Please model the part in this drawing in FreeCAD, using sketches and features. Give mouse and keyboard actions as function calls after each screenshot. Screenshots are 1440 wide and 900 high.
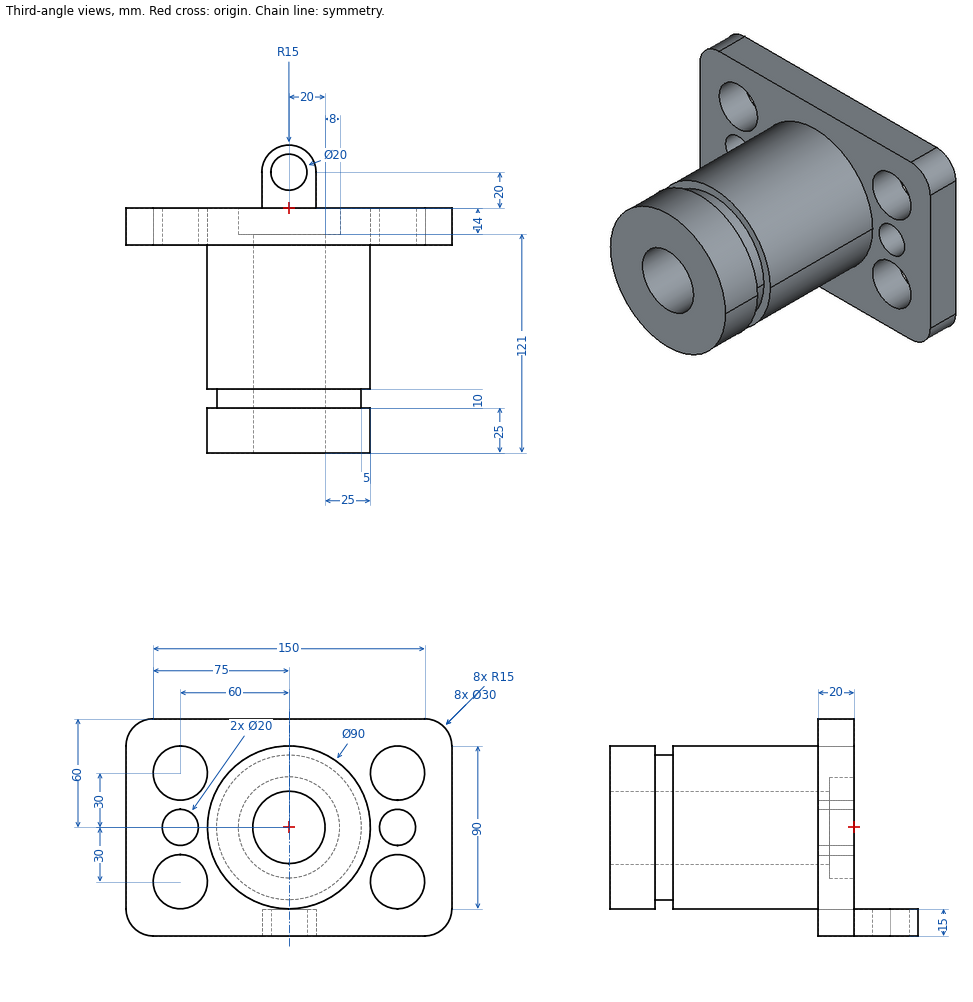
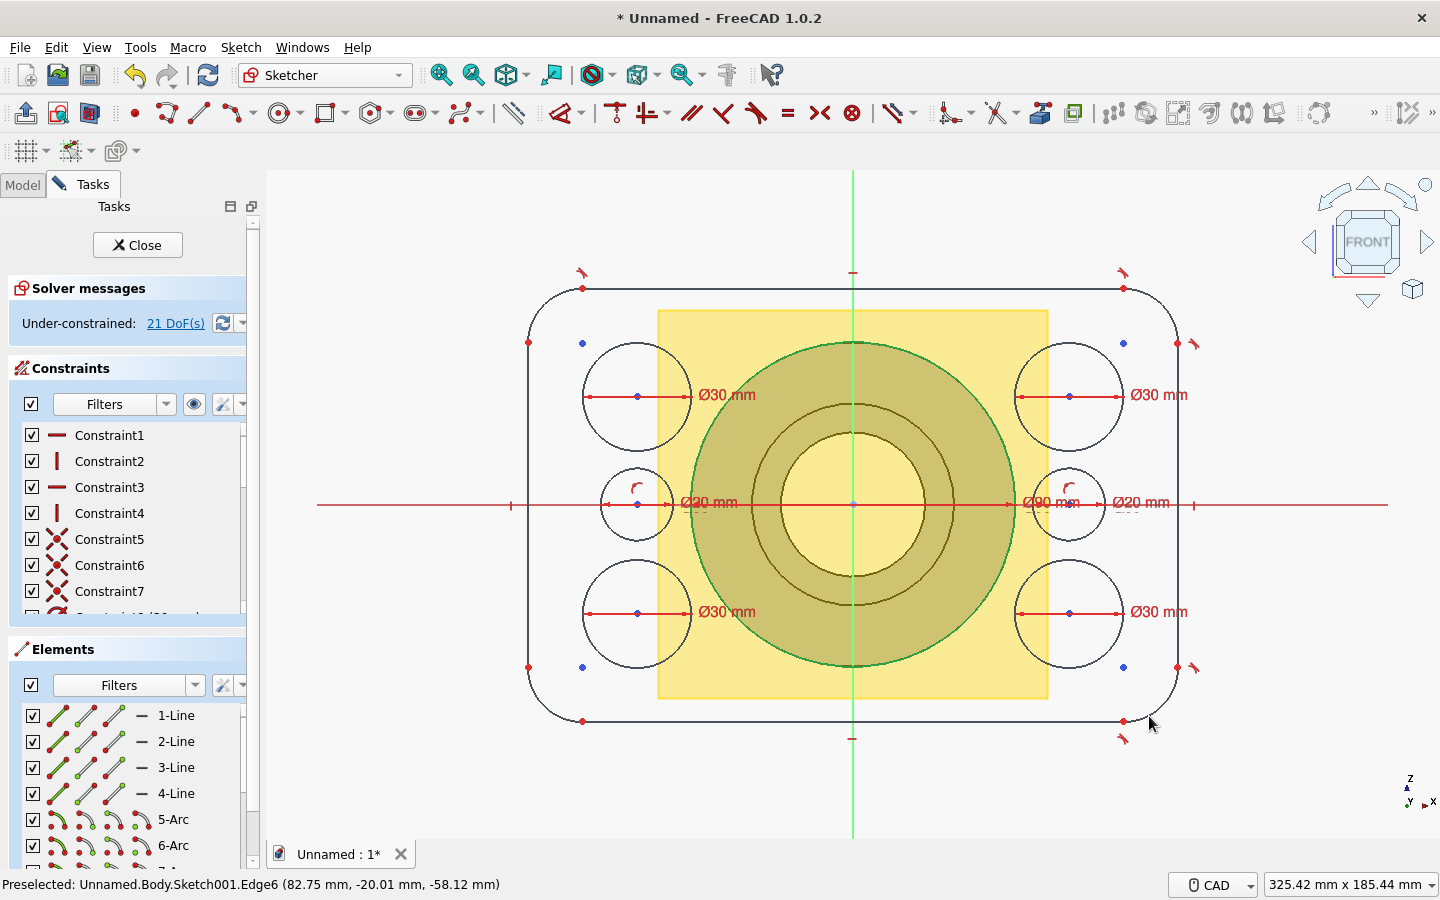
click(961, 722)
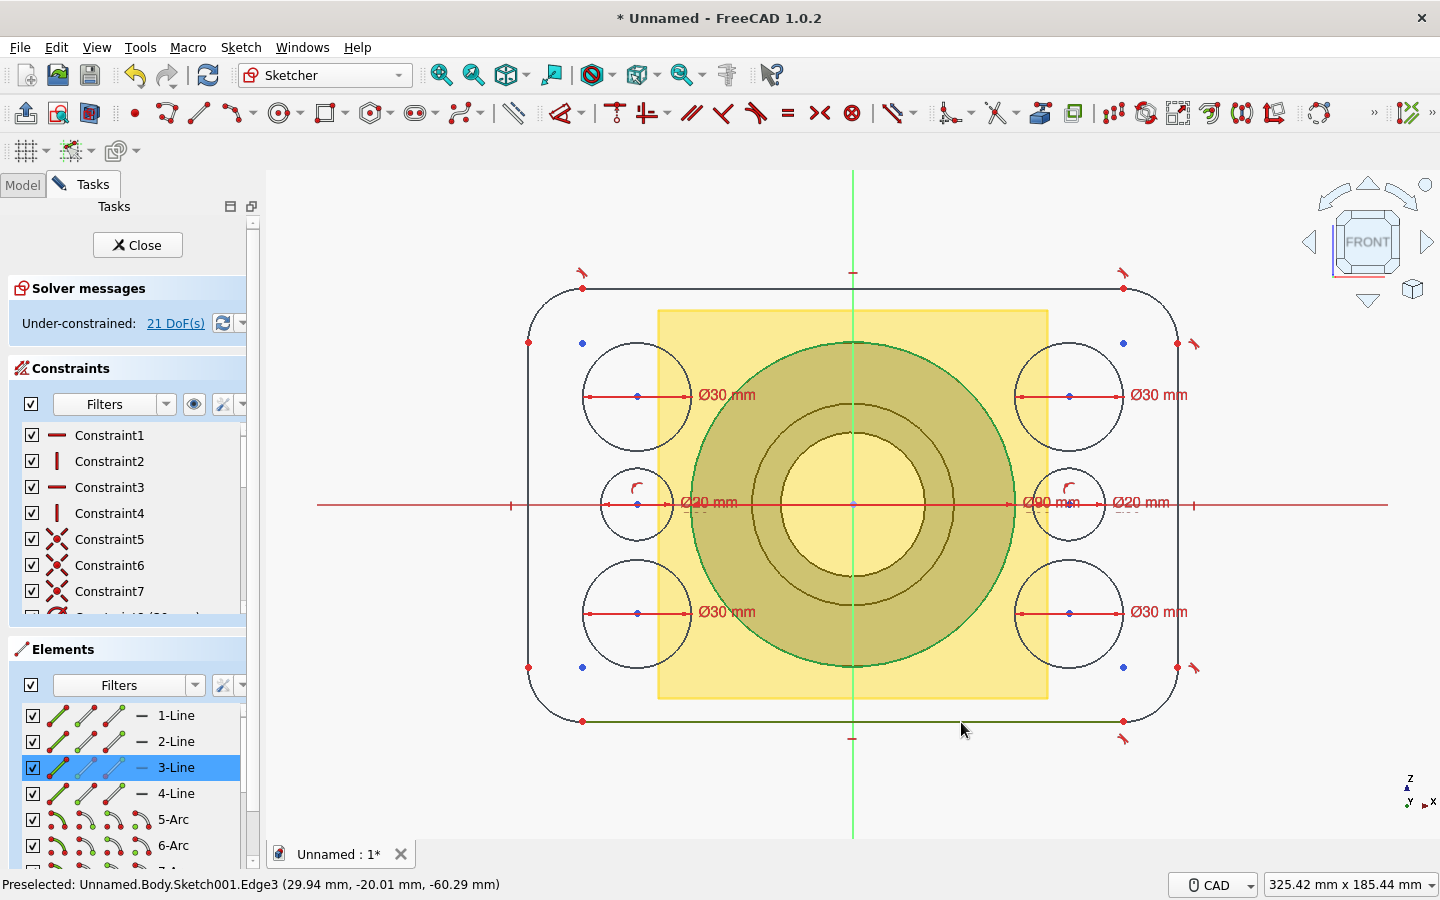
click(534, 692)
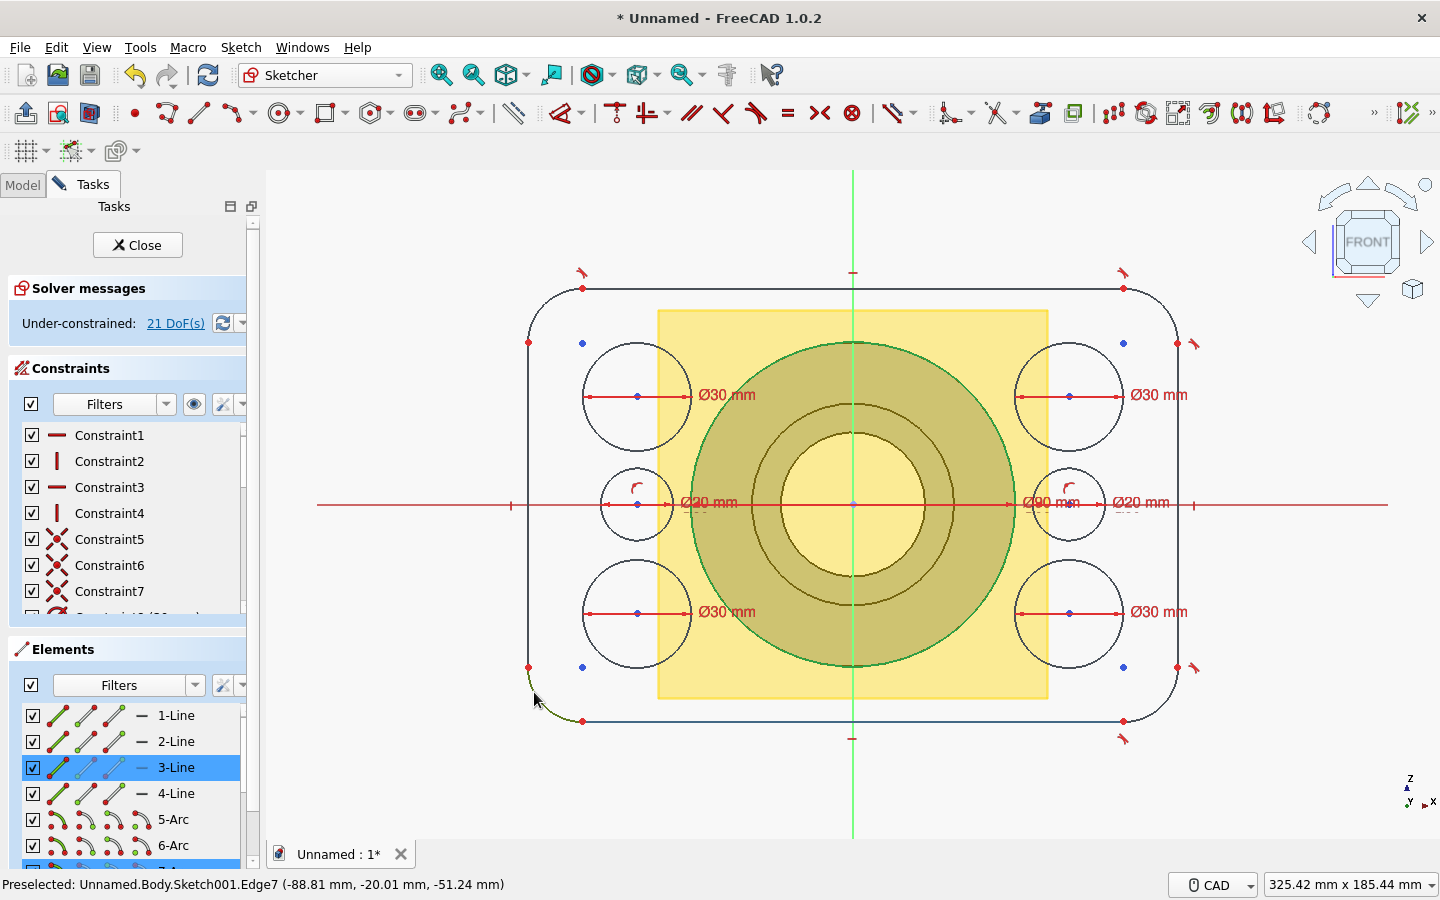
click(756, 114)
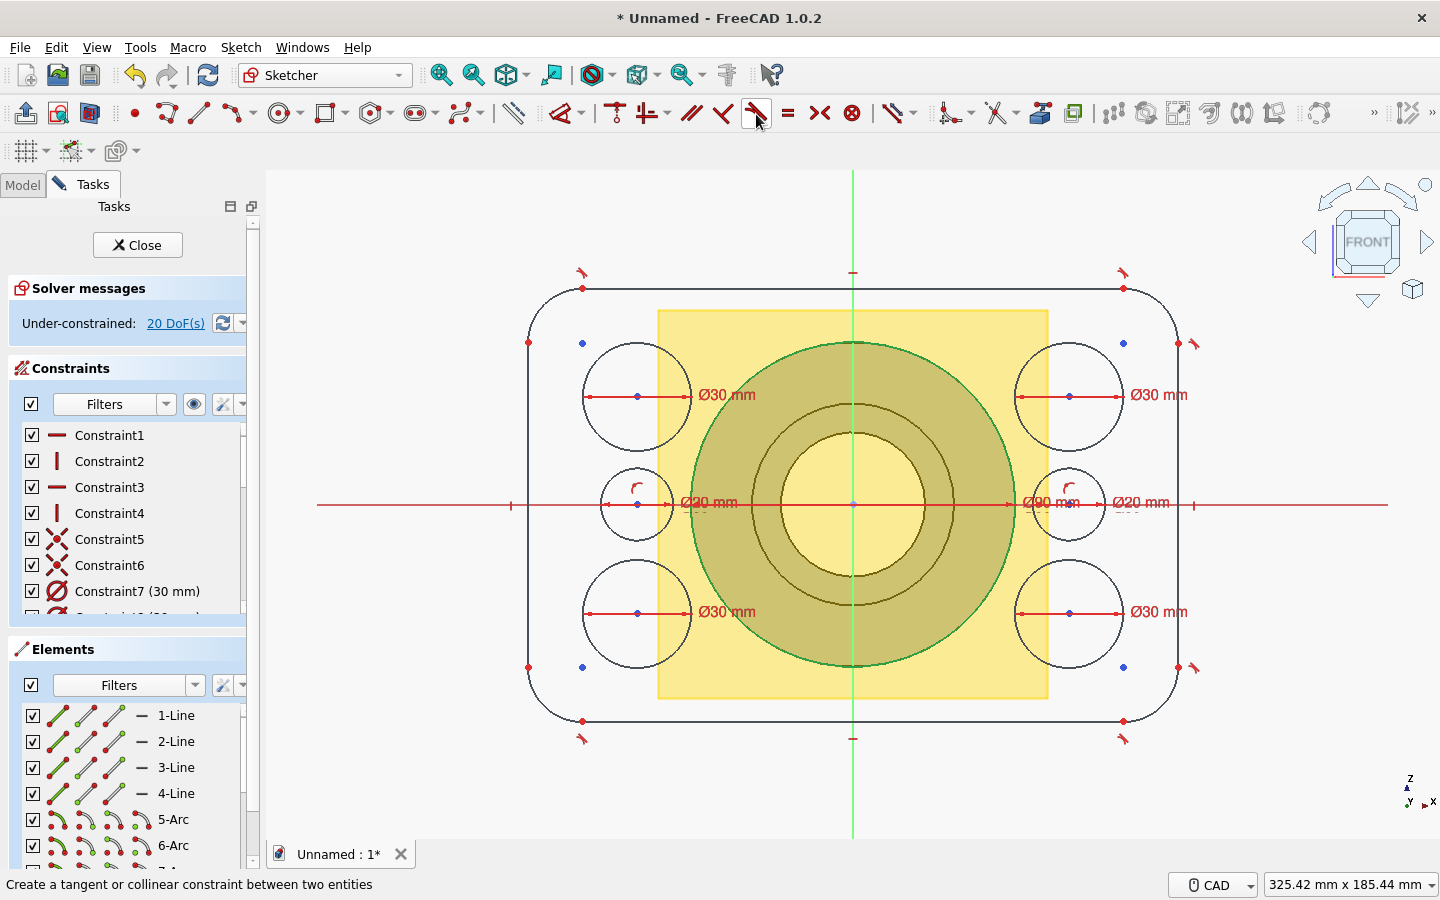
click(528, 570)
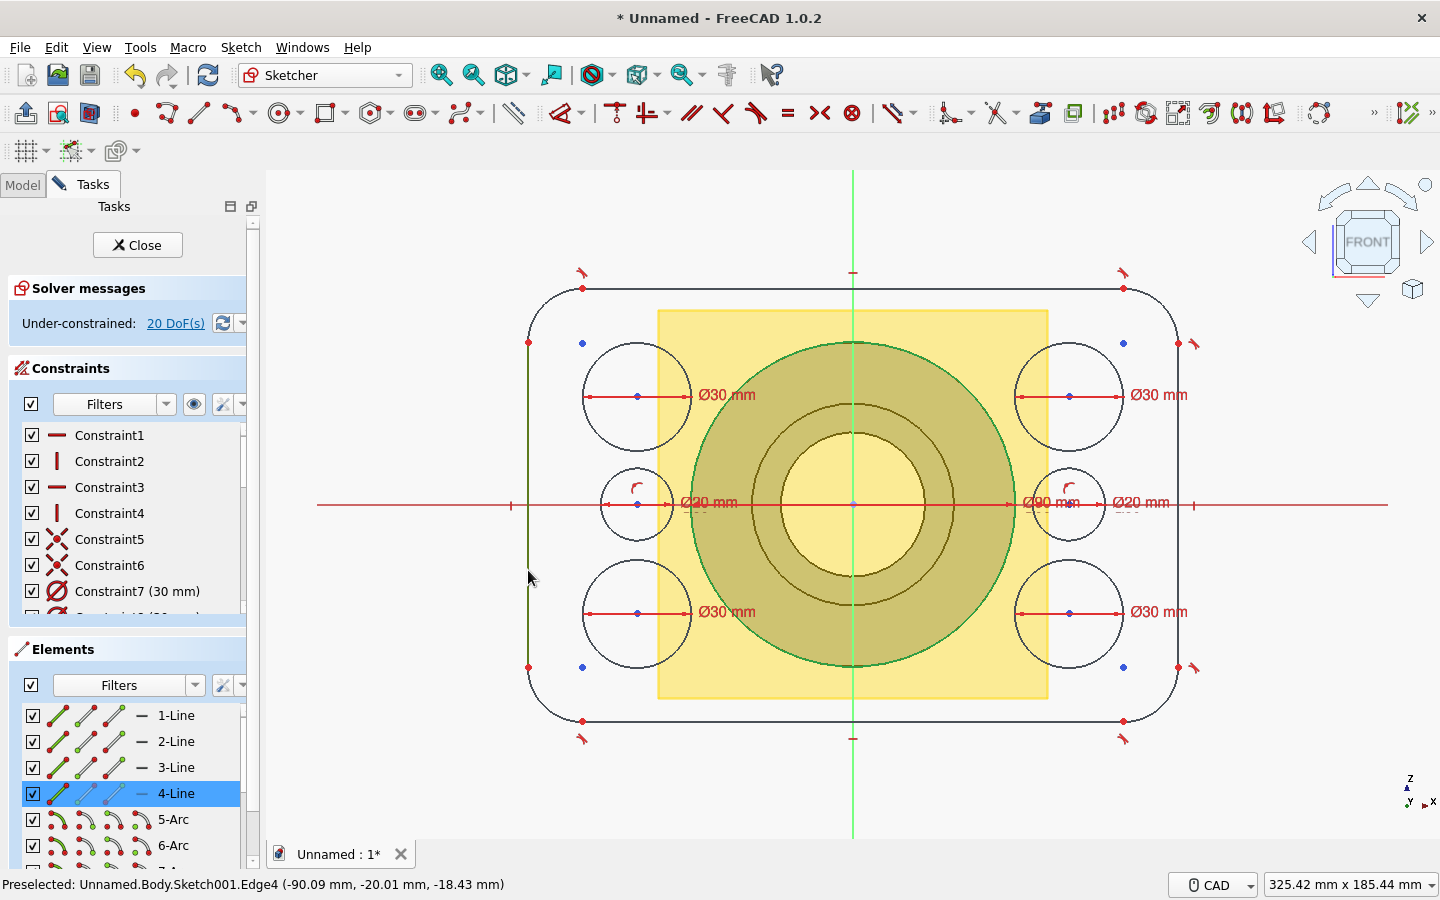
click(534, 693)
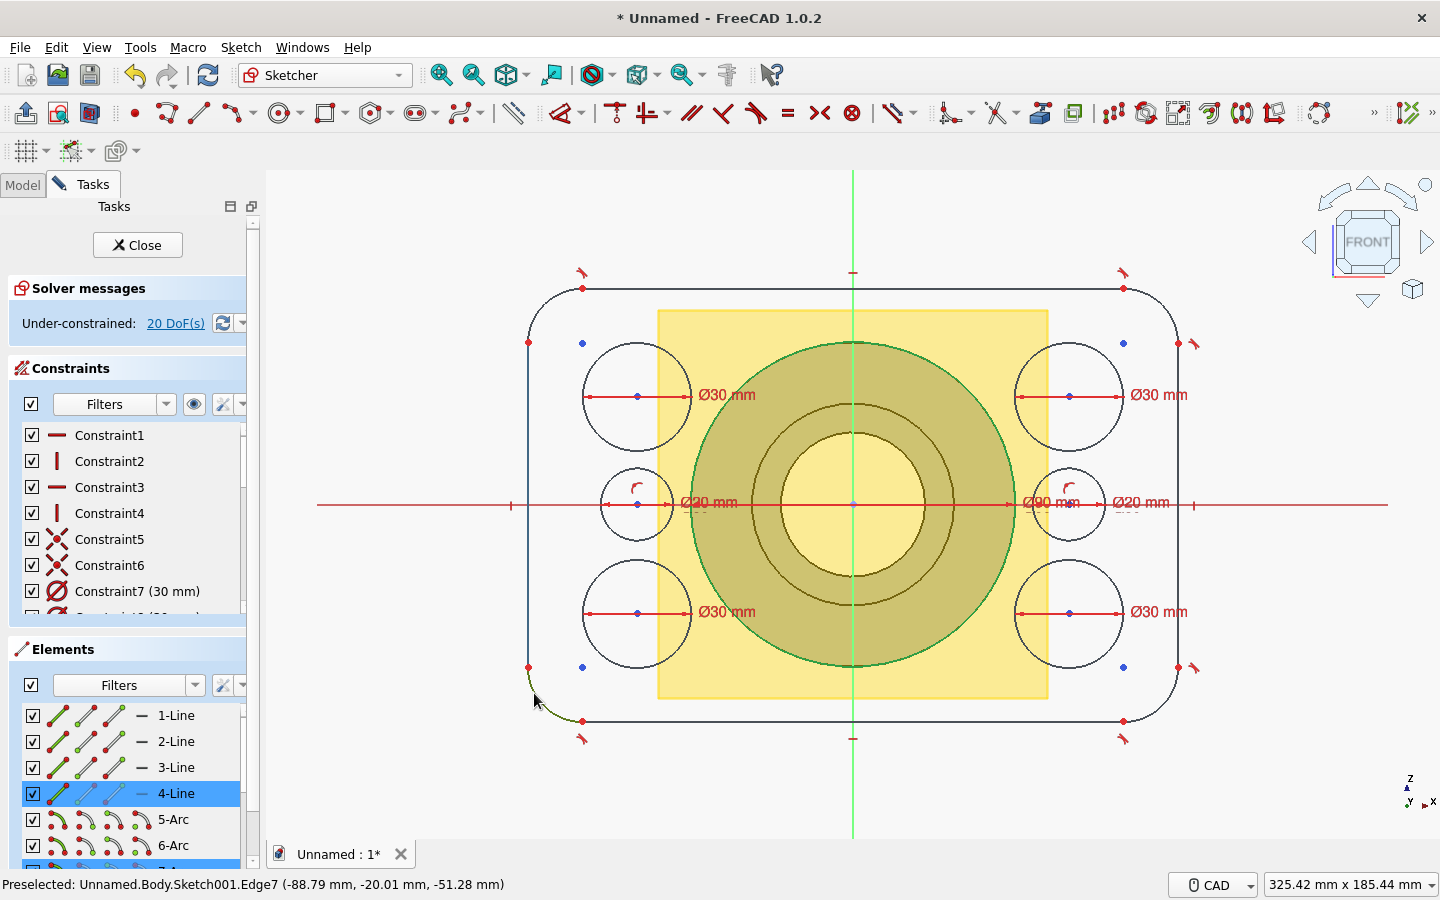
key(t)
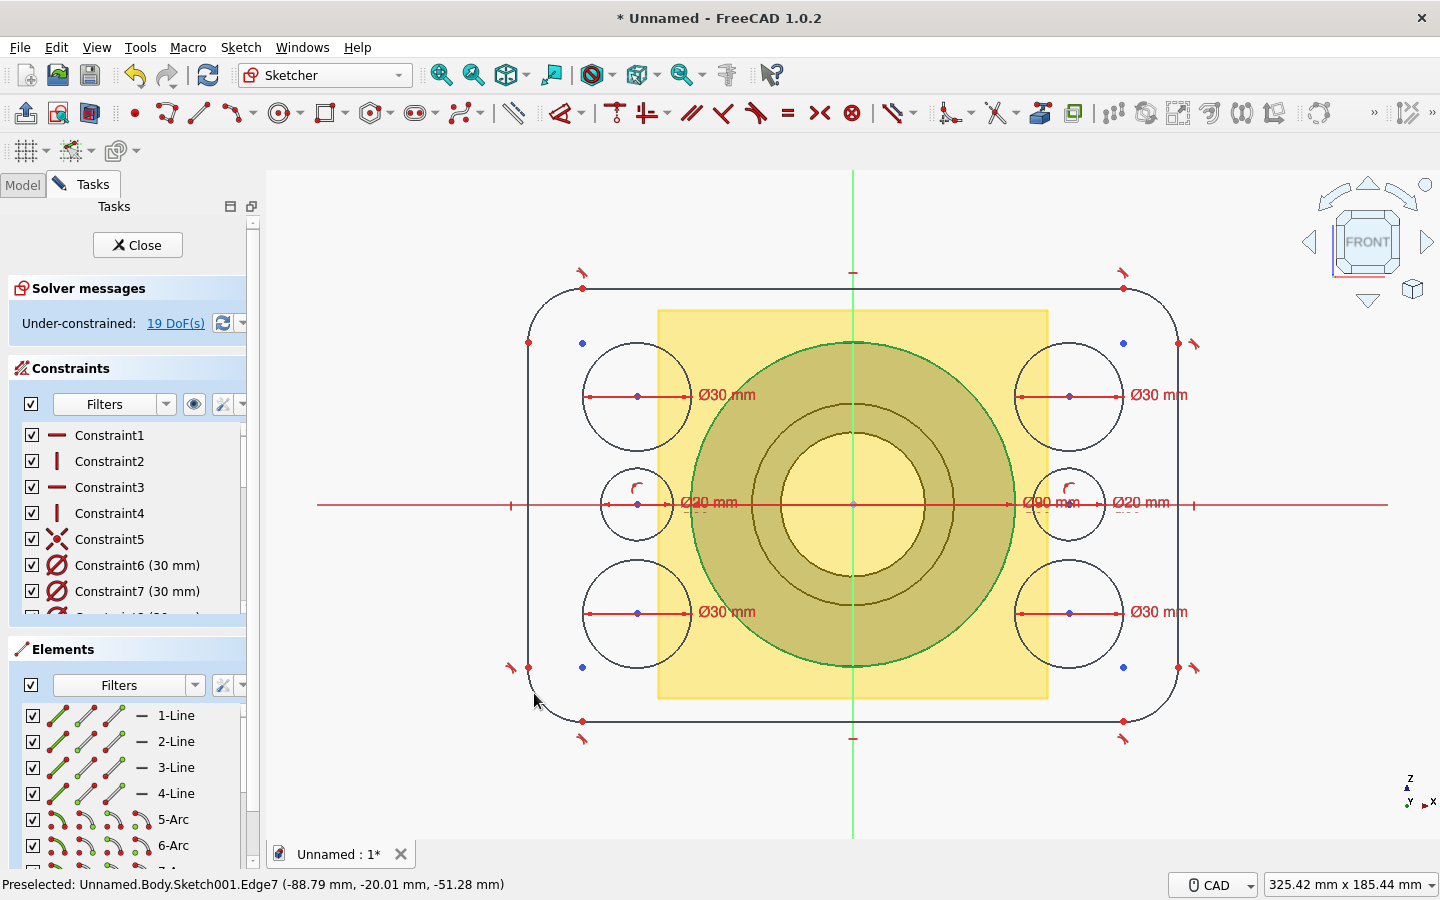
click(528, 570)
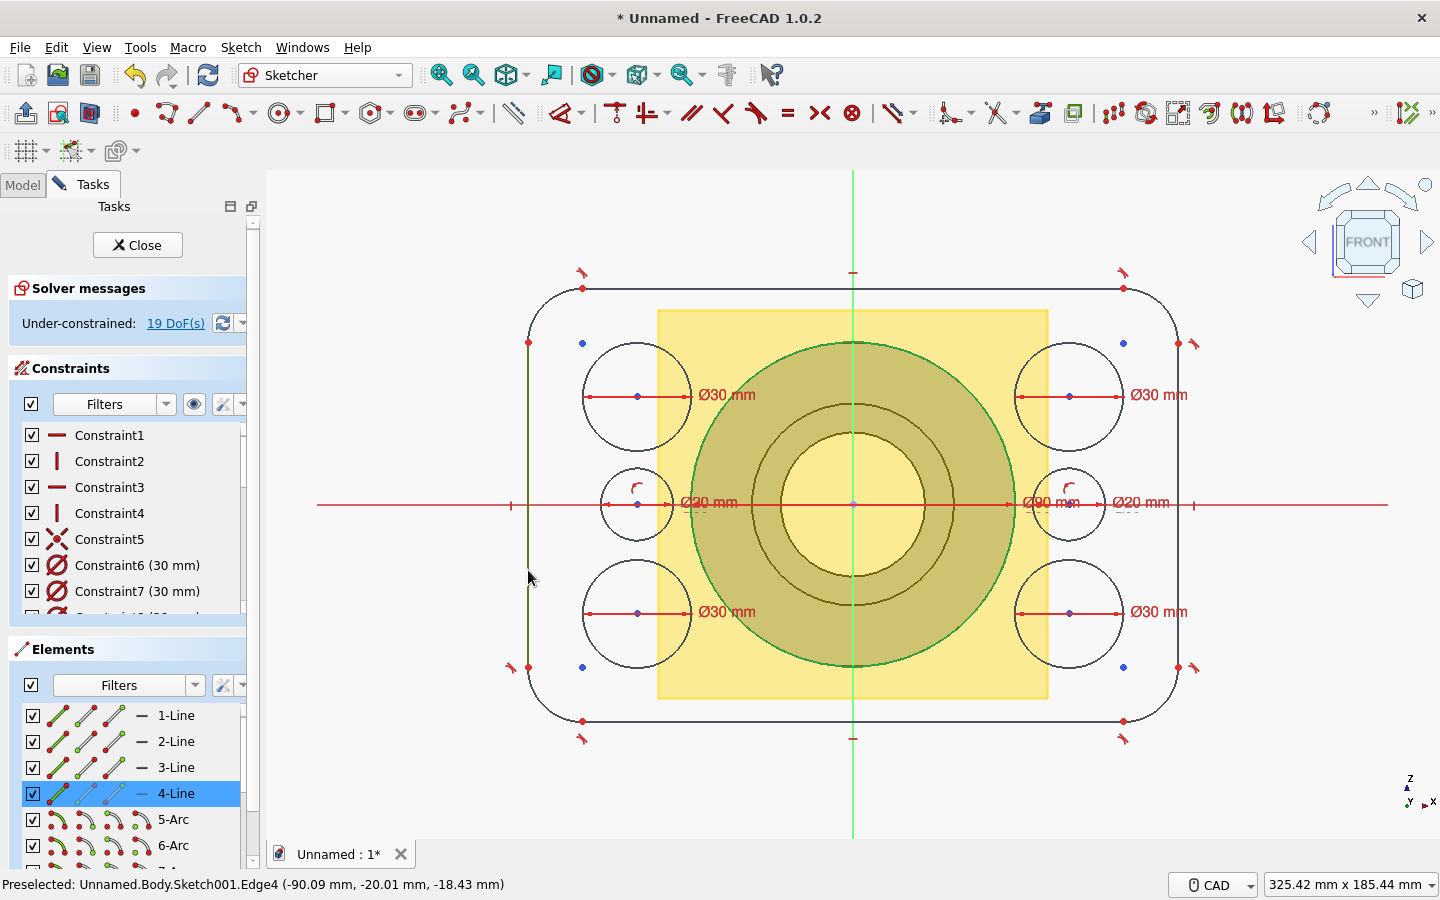
click(558, 295)